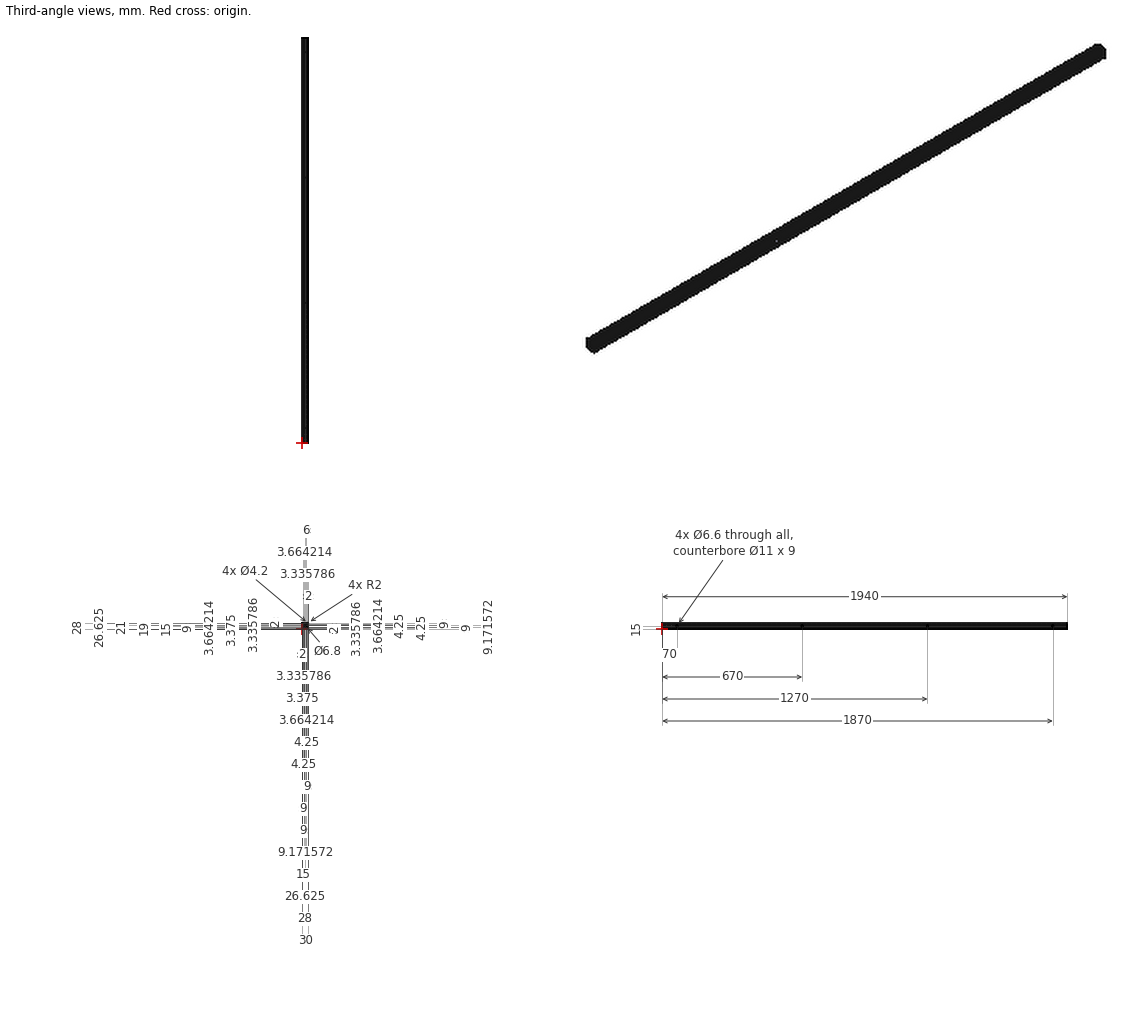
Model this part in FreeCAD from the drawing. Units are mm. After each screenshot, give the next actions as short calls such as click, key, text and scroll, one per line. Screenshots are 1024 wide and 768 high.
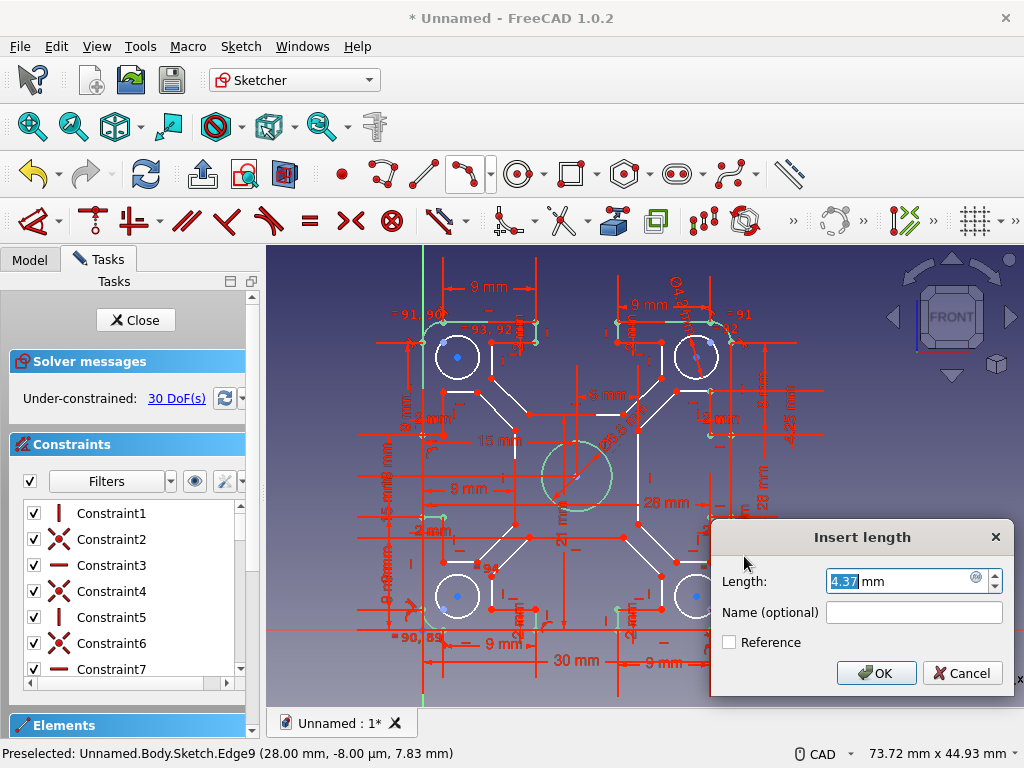
text(4.25)
key(Return)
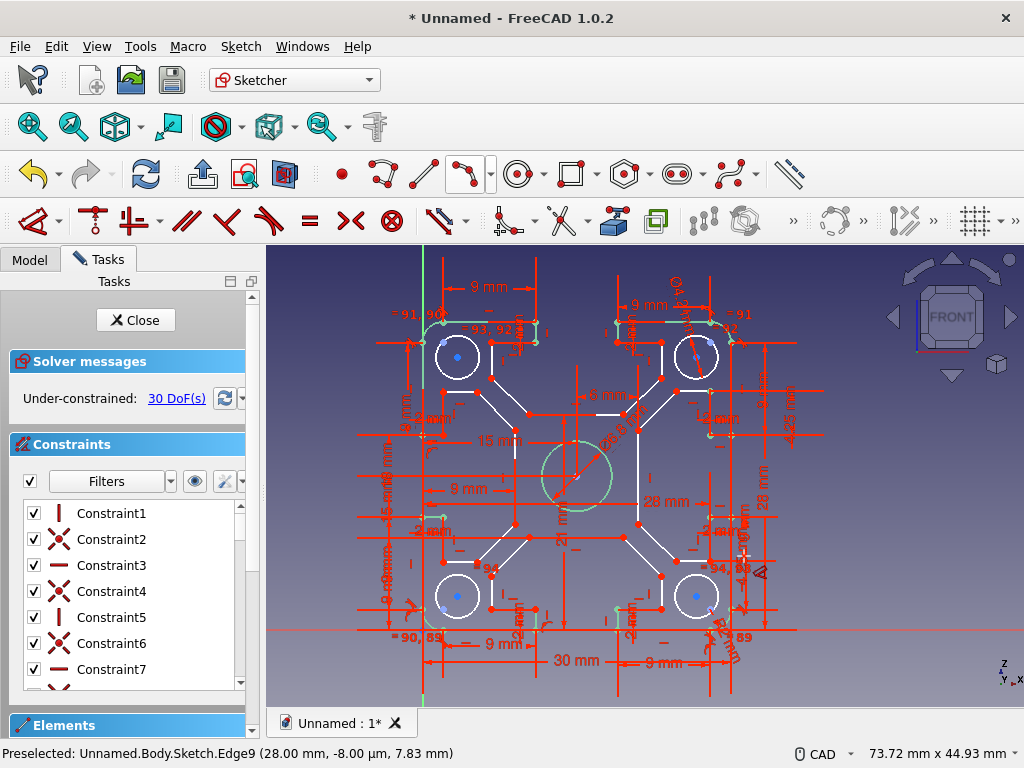
click(631, 610)
click(640, 644)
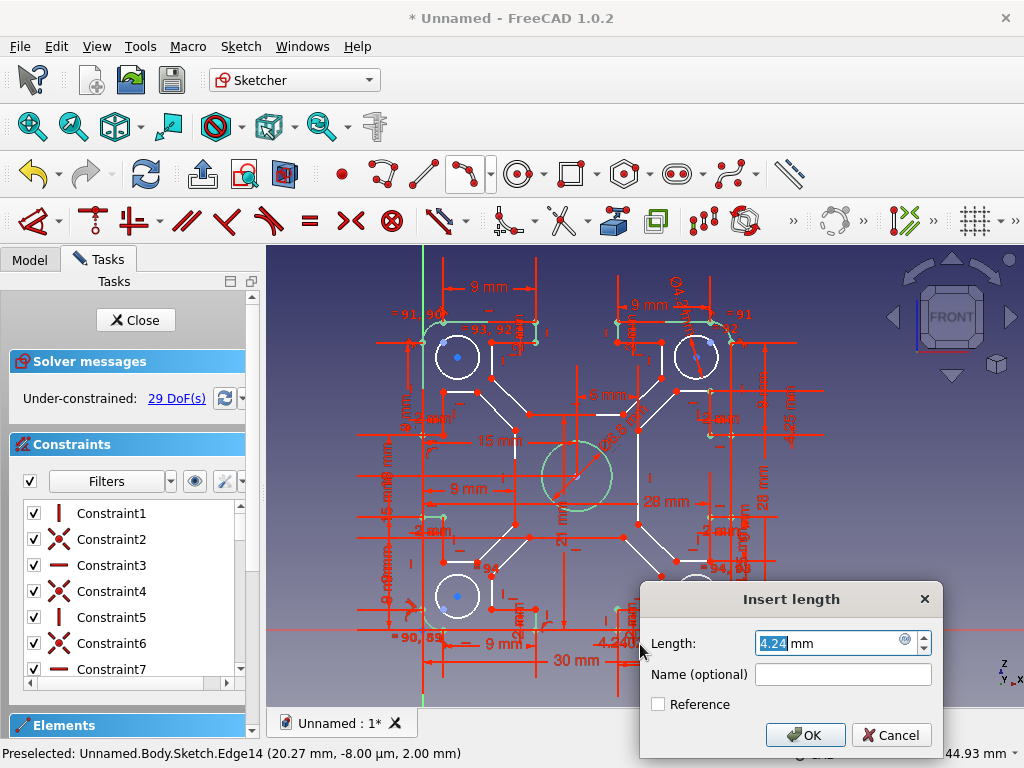
text(4.25)
key(Return)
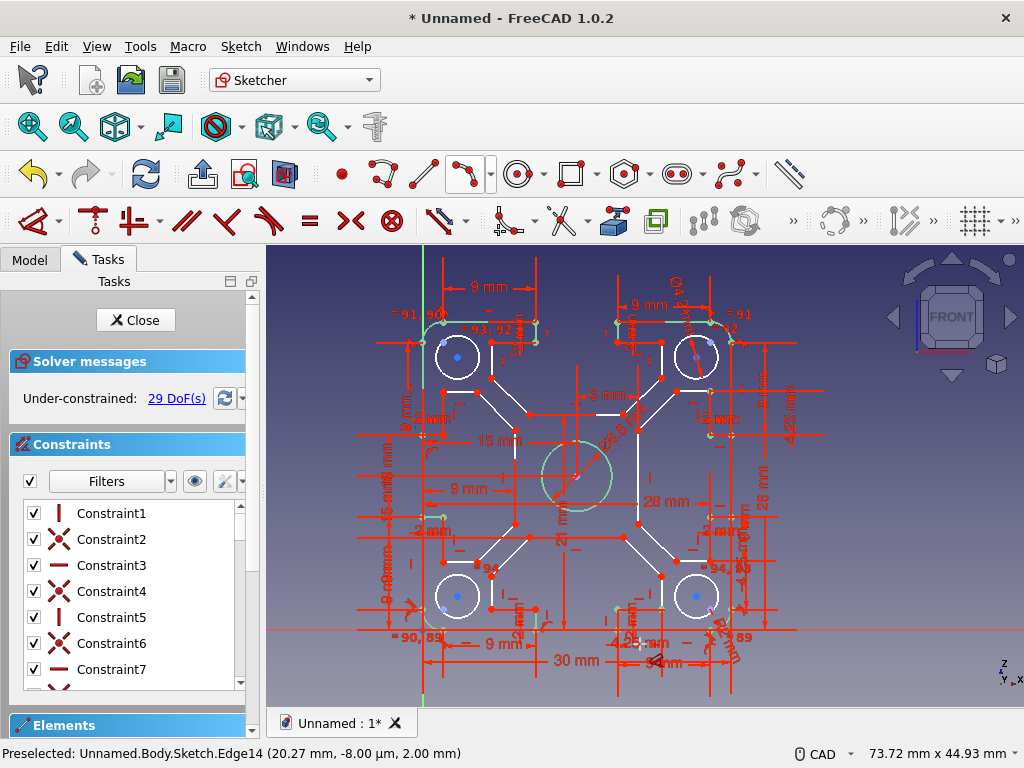
click(505, 610)
click(514, 576)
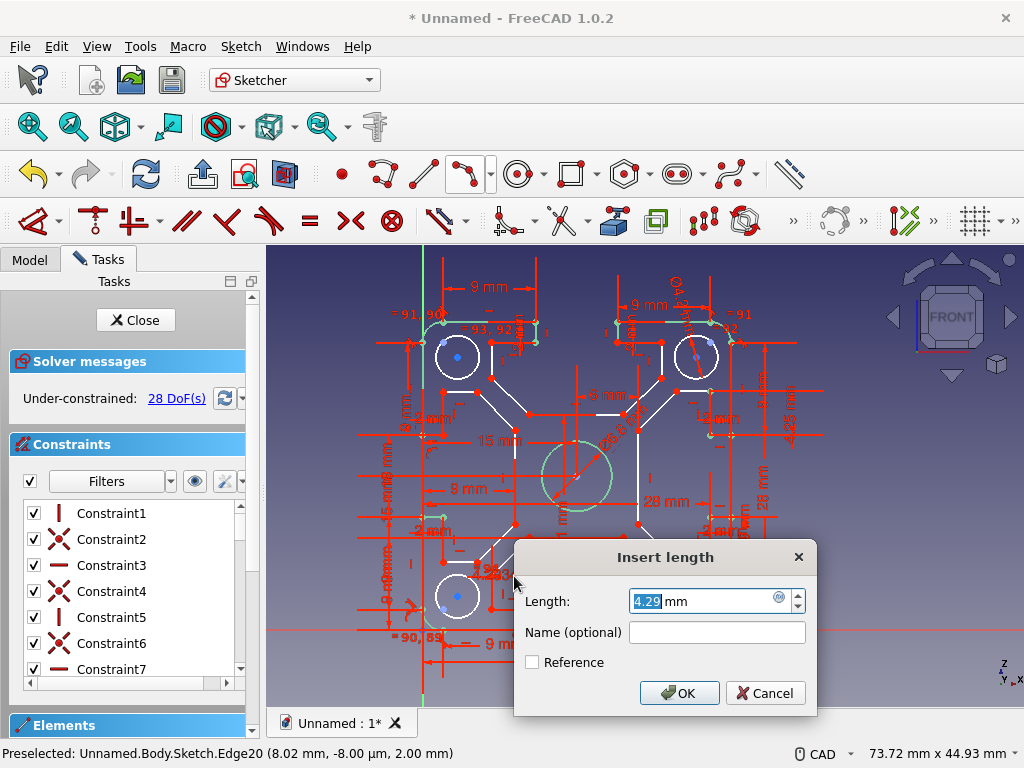
text(4.25)
key(Return)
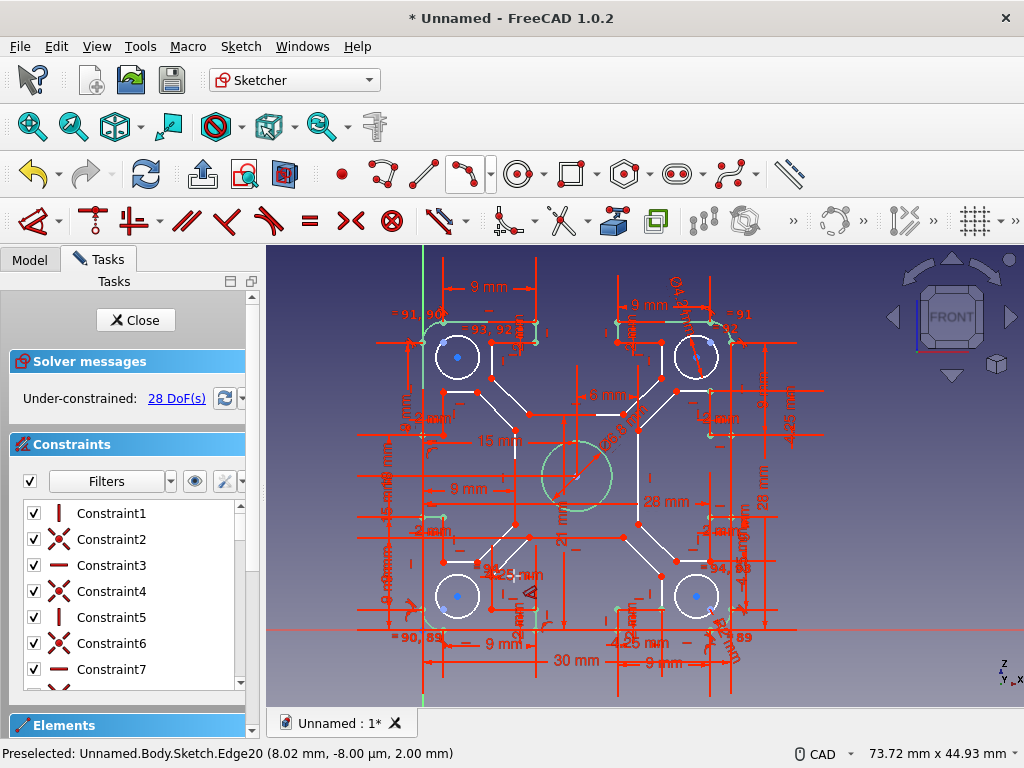
click(443, 531)
click(361, 540)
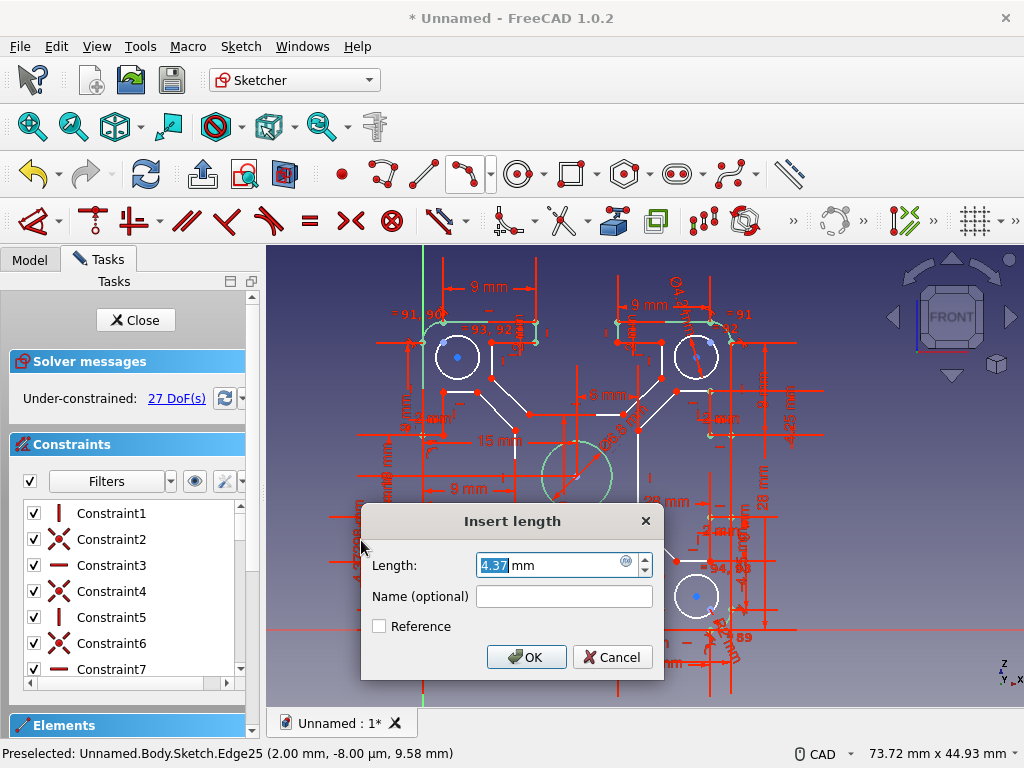
text(4.25)
key(Return)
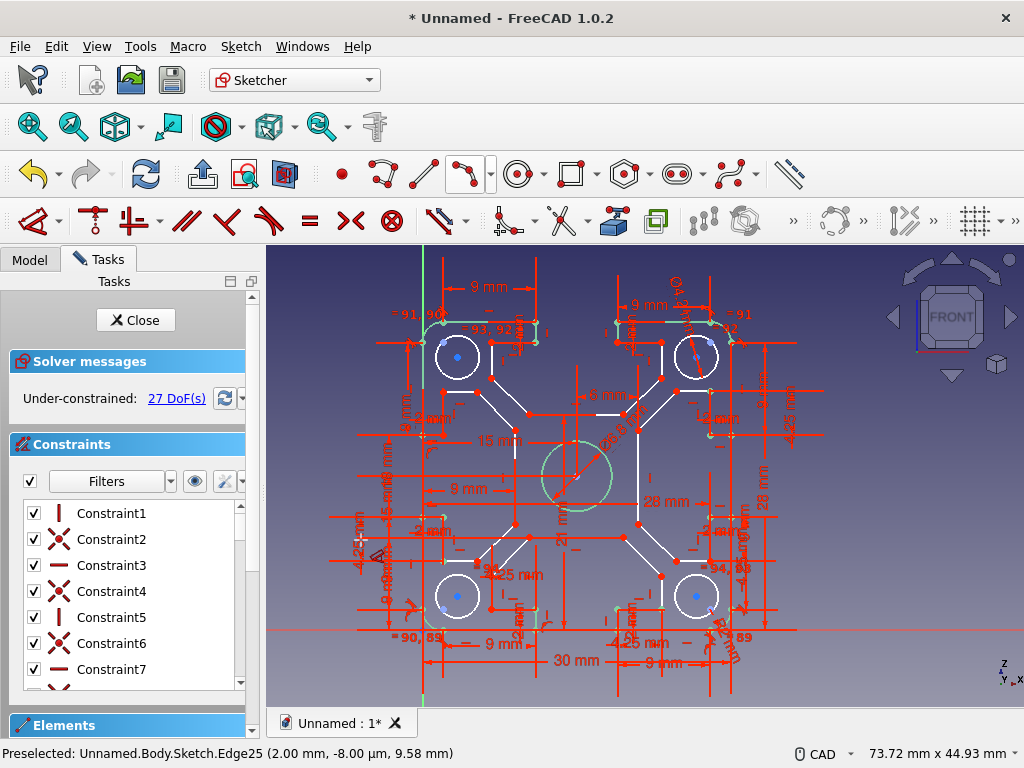
click(443, 405)
click(337, 414)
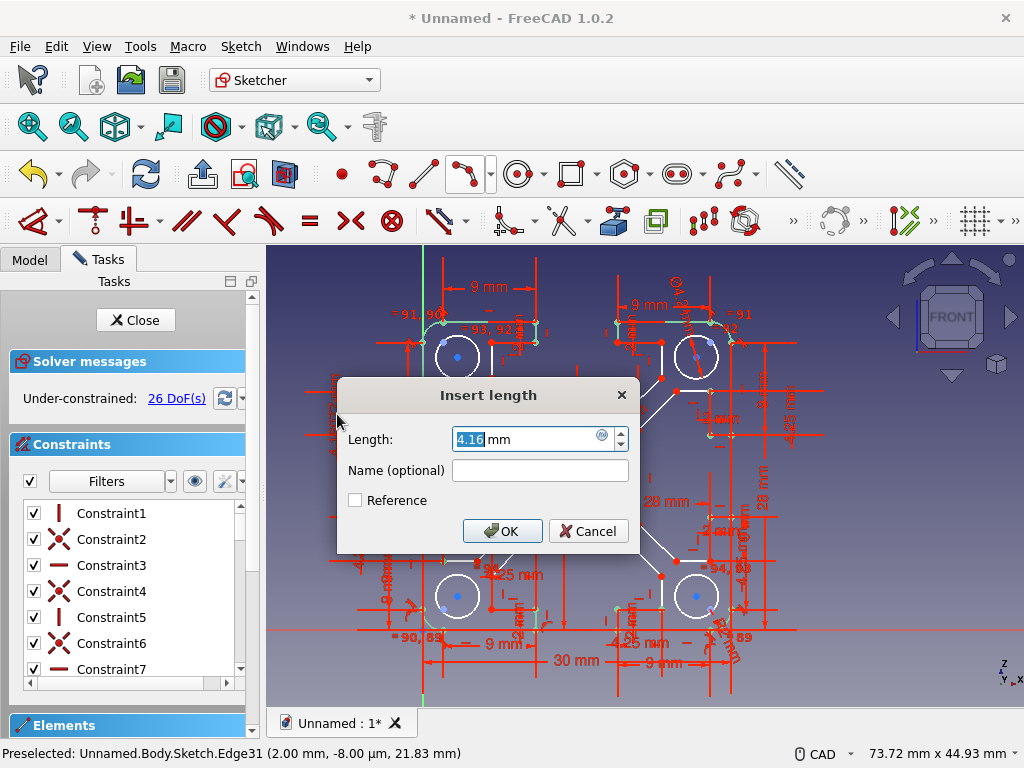
text(4.25)
key(Return)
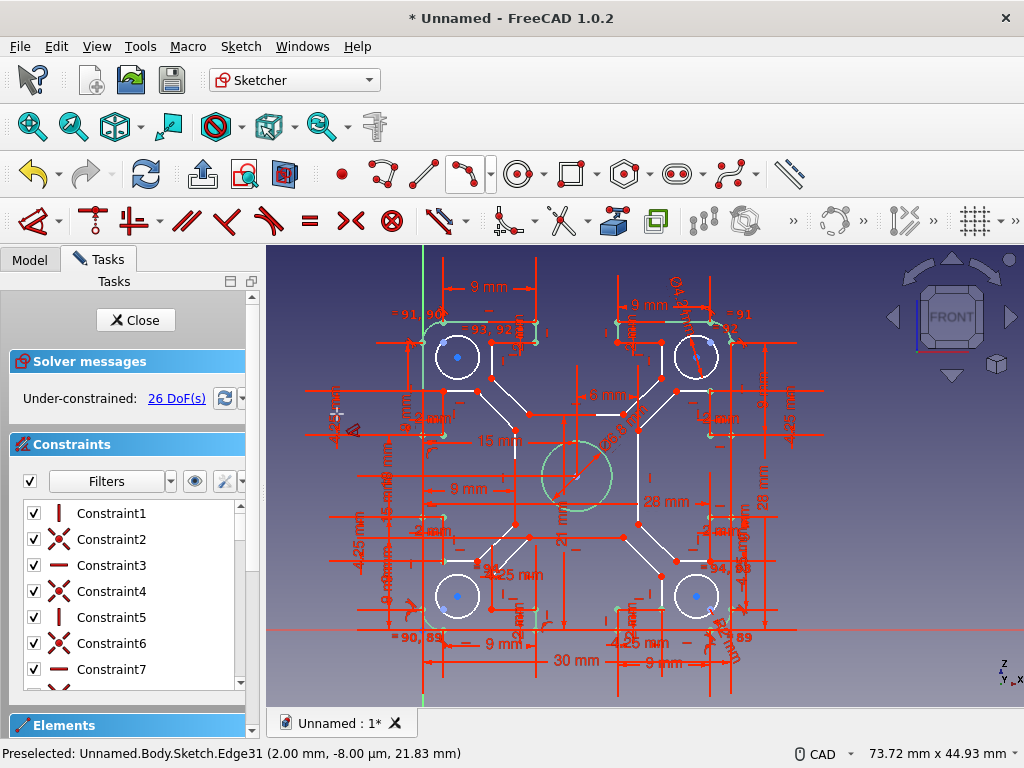
click(522, 343)
click(514, 309)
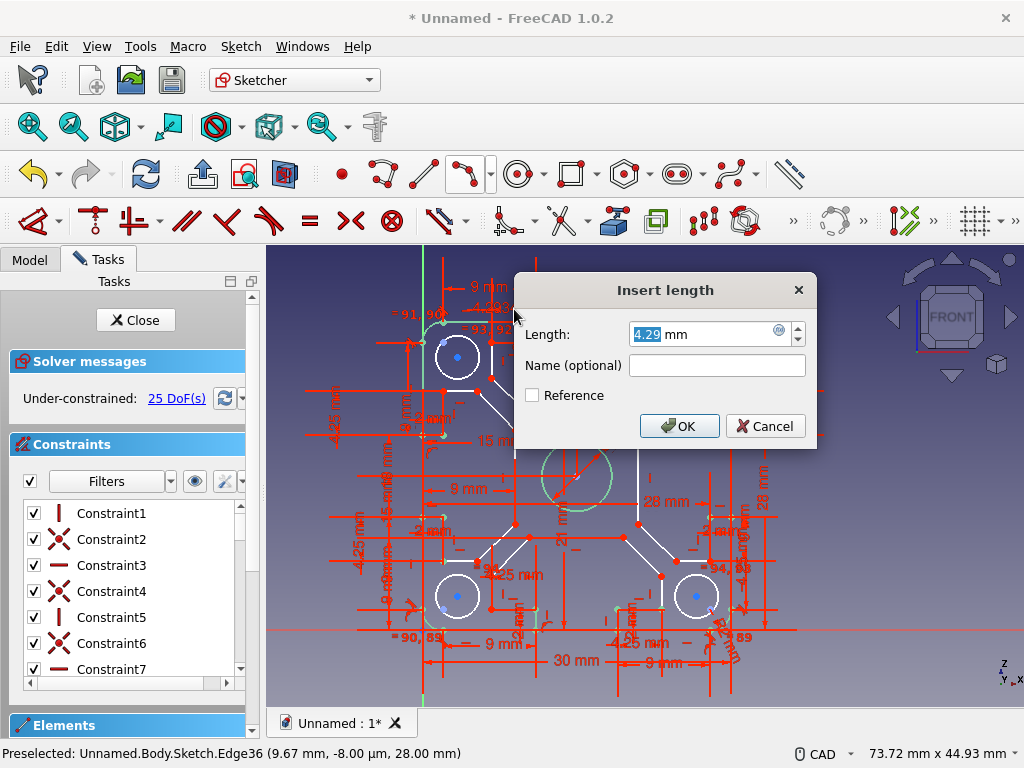
text(4.25)
key(Return)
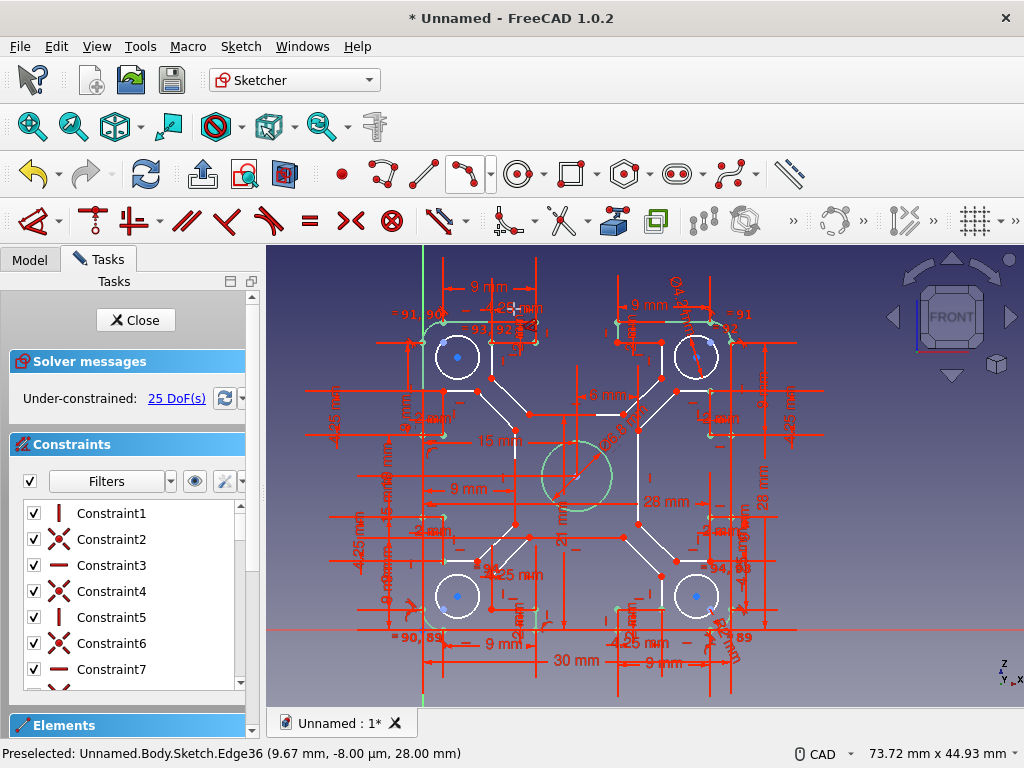
click(648, 343)
click(640, 285)